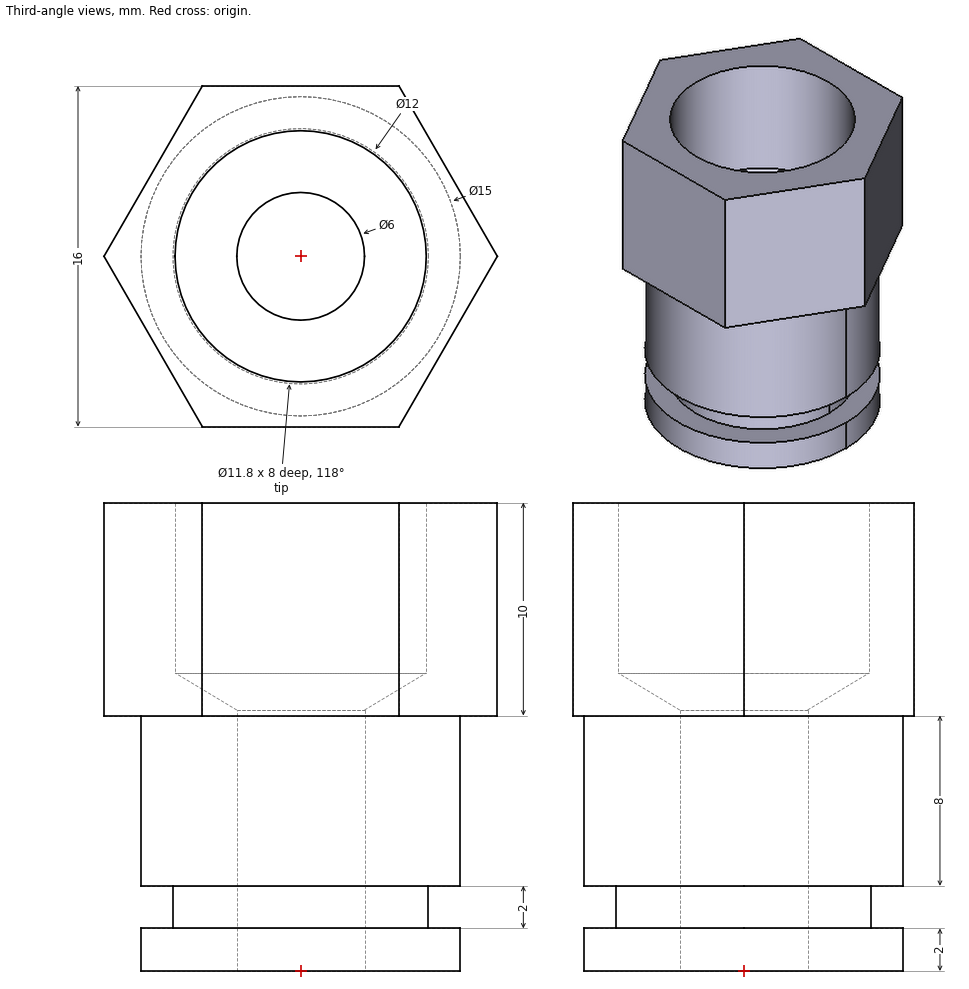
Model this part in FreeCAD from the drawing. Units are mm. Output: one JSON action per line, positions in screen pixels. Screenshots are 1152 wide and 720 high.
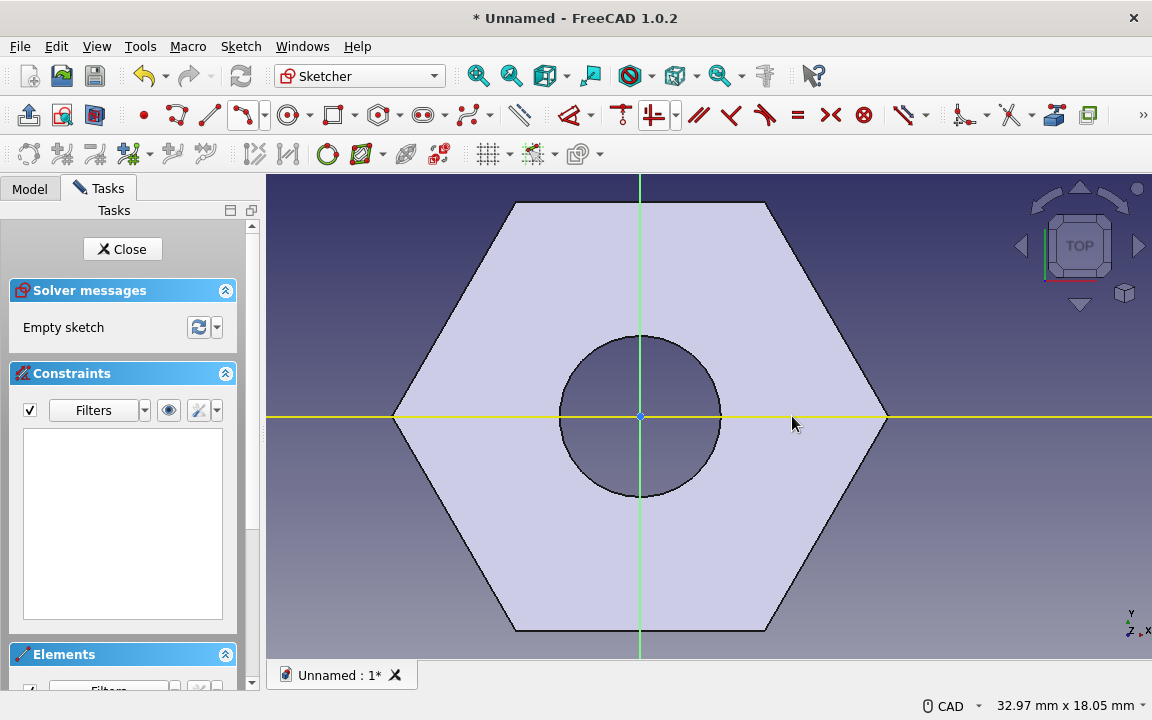
{"action": "left_click", "coordinate": [288, 116]}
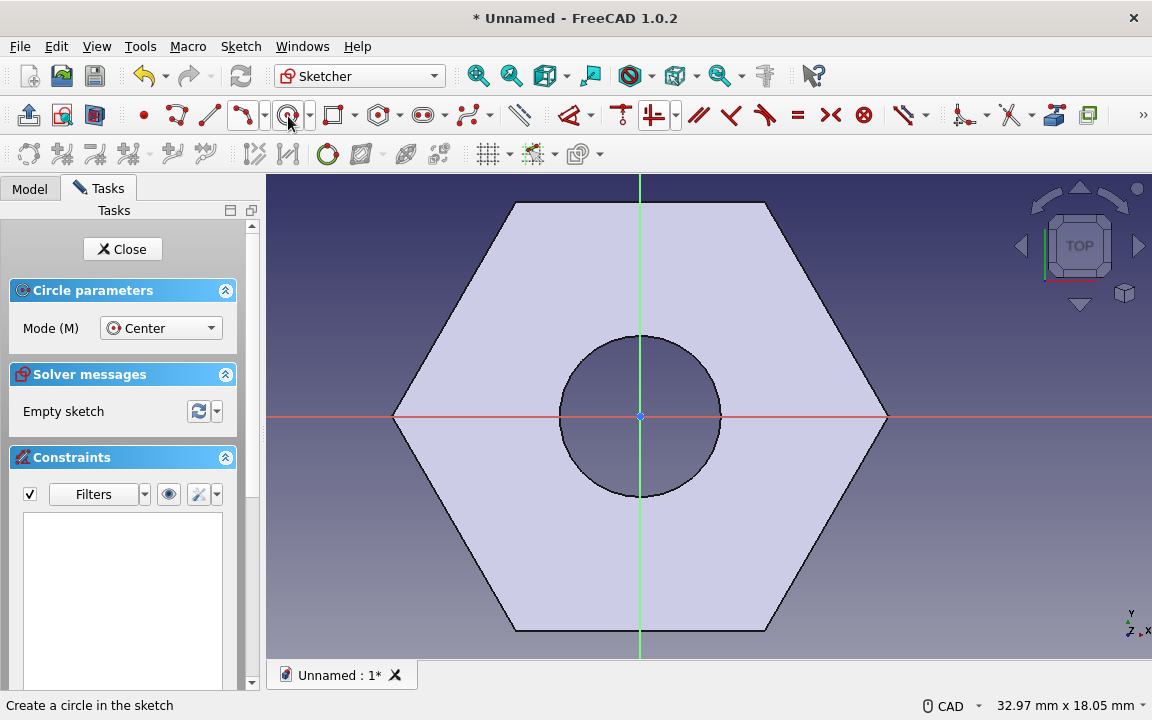
{"action": "left_click", "coordinate": [640, 416]}
{"action": "left_click", "coordinate": [752, 304]}
{"action": "key", "text": "Escape"}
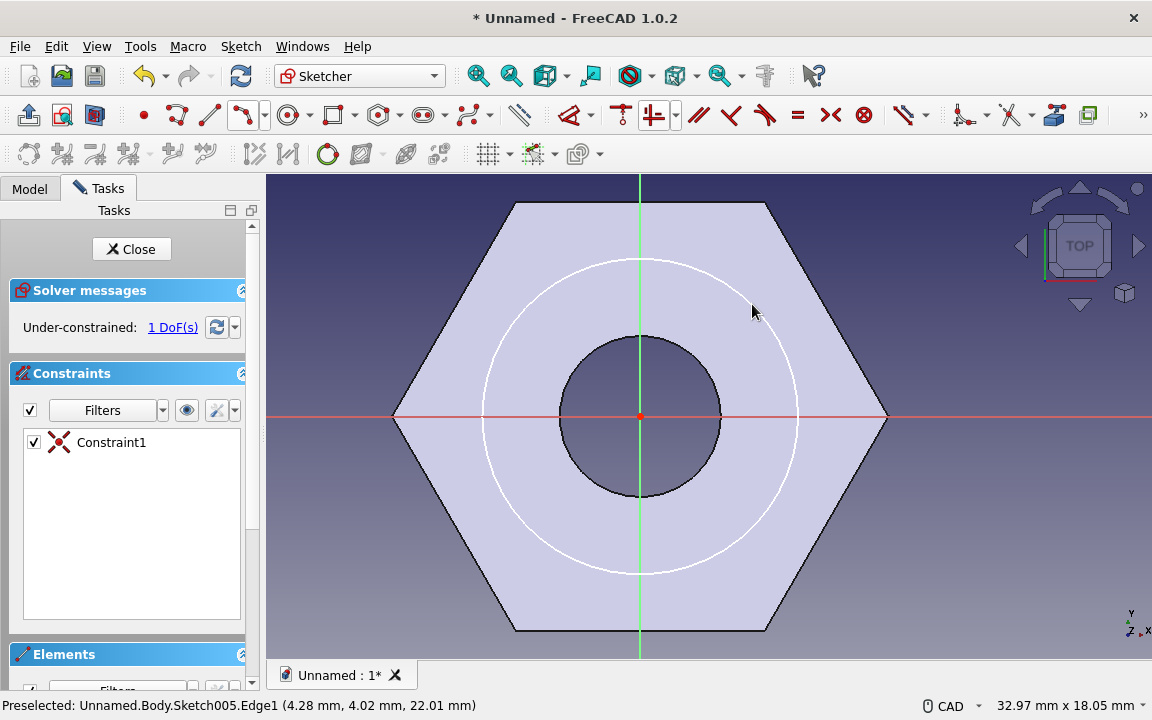
{"action": "key", "text": "d"}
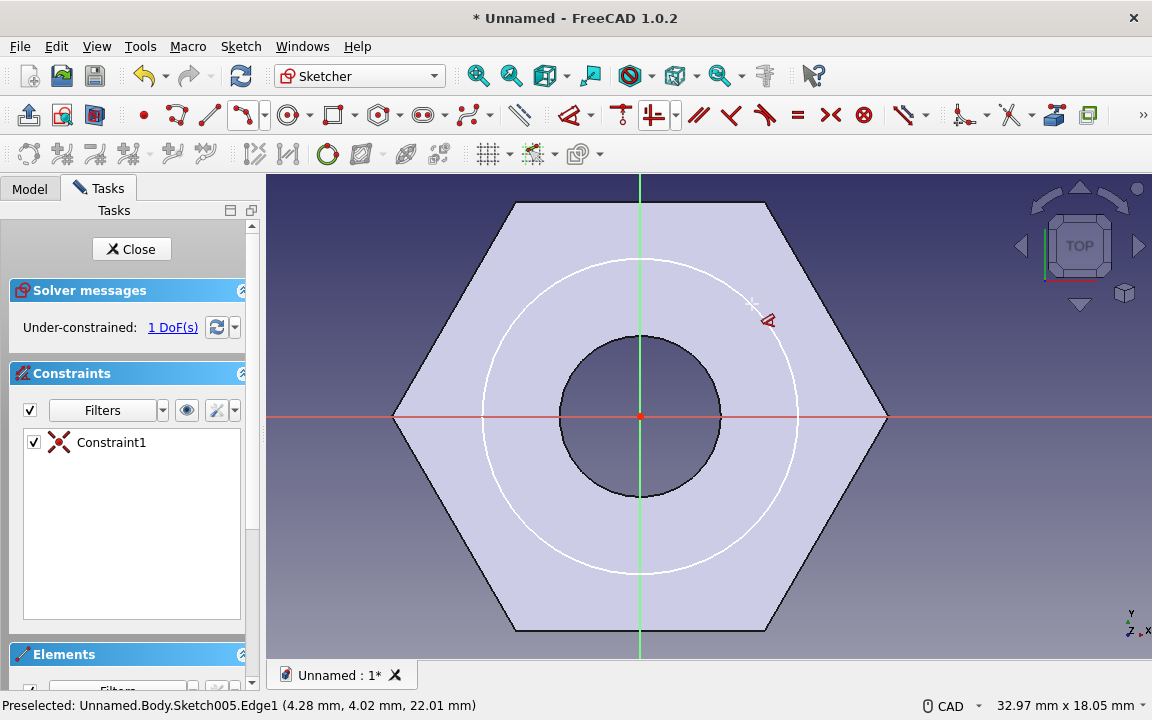
{"action": "left_click", "coordinate": [752, 305]}
{"action": "left_click", "coordinate": [775, 282]}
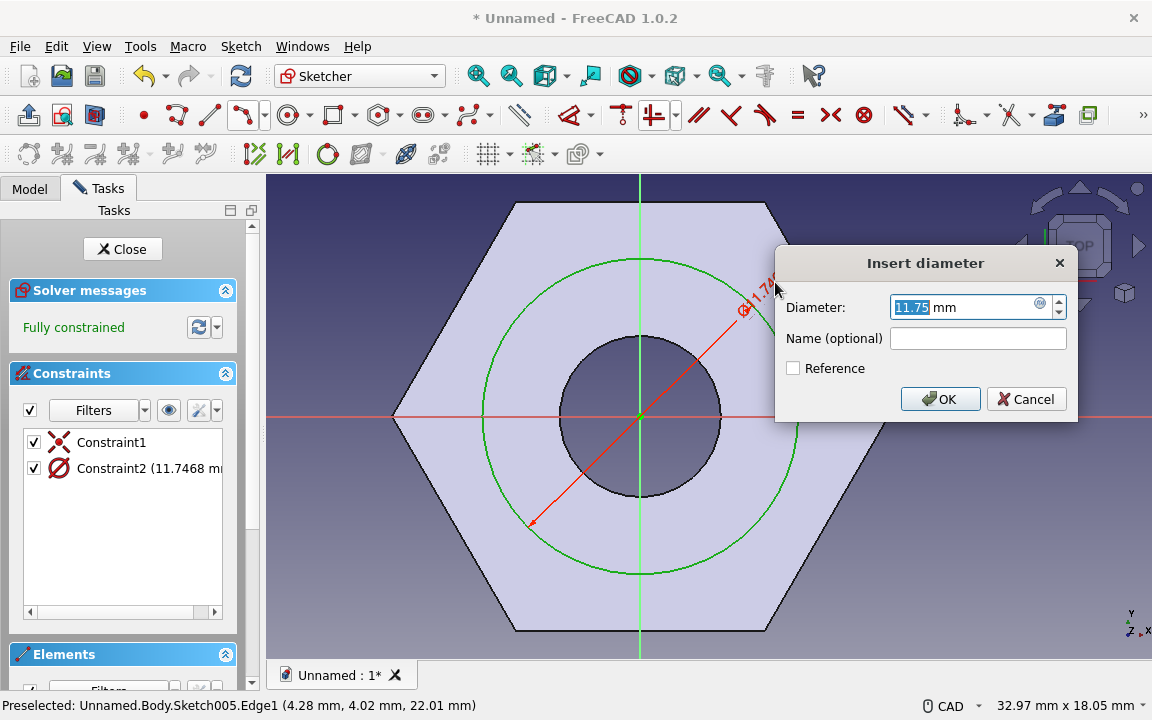
{"action": "type", "text": "11.8"}
{"action": "key", "text": "Return"}
{"action": "key", "text": "Escape"}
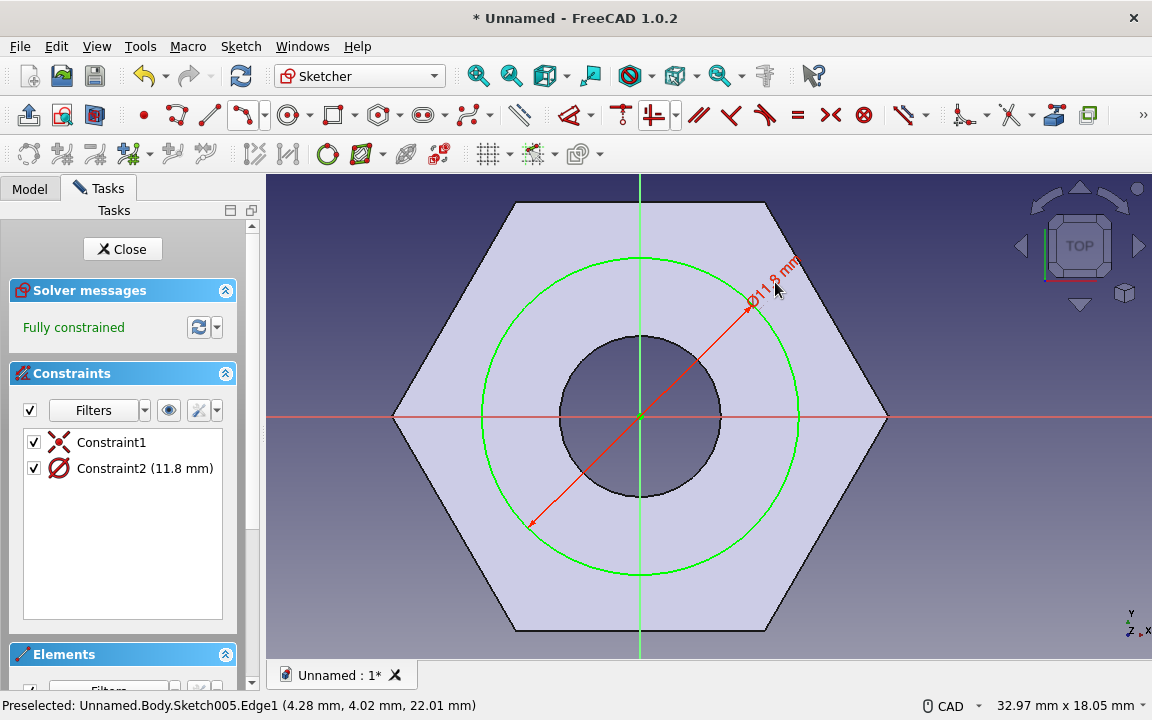
{"action": "left_click", "coordinate": [123, 249]}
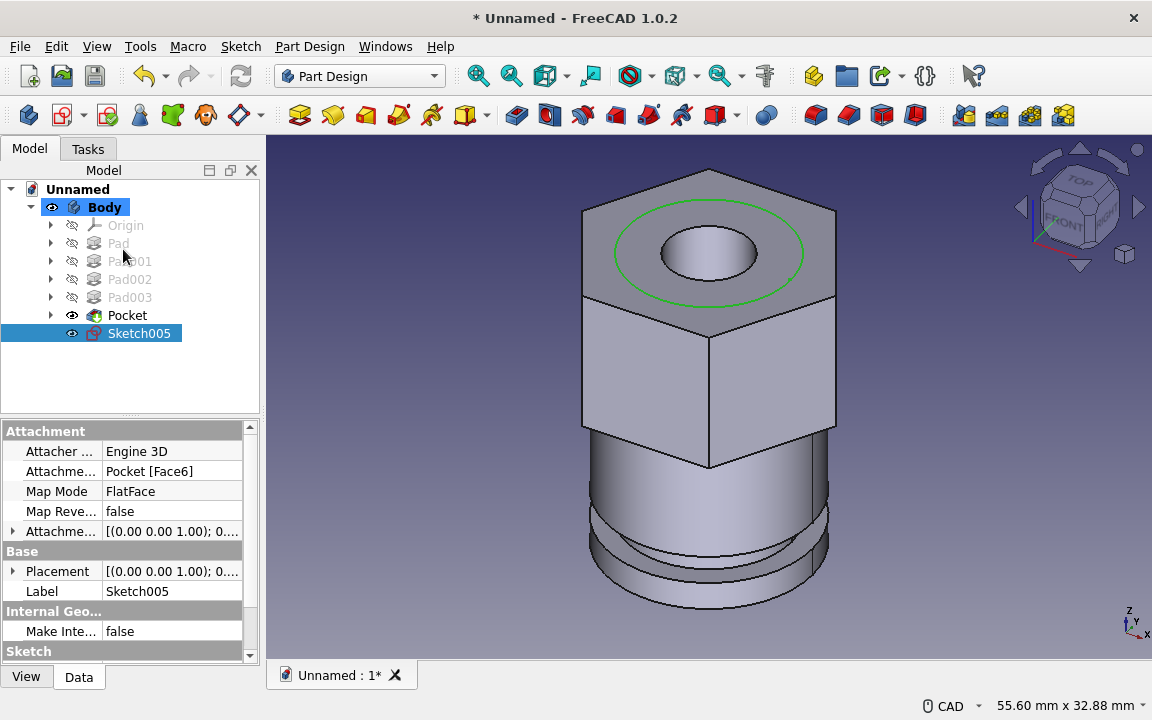
{"action": "left_click", "coordinate": [550, 116]}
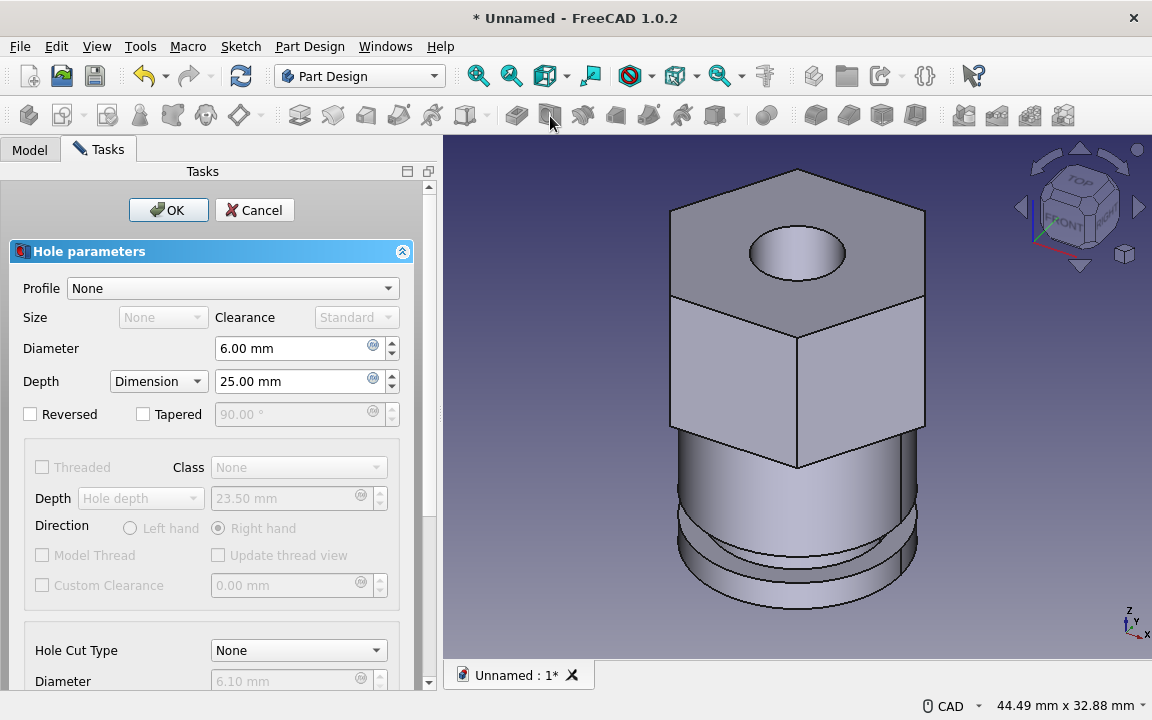
{"action": "triple_click", "coordinate": [300, 348]}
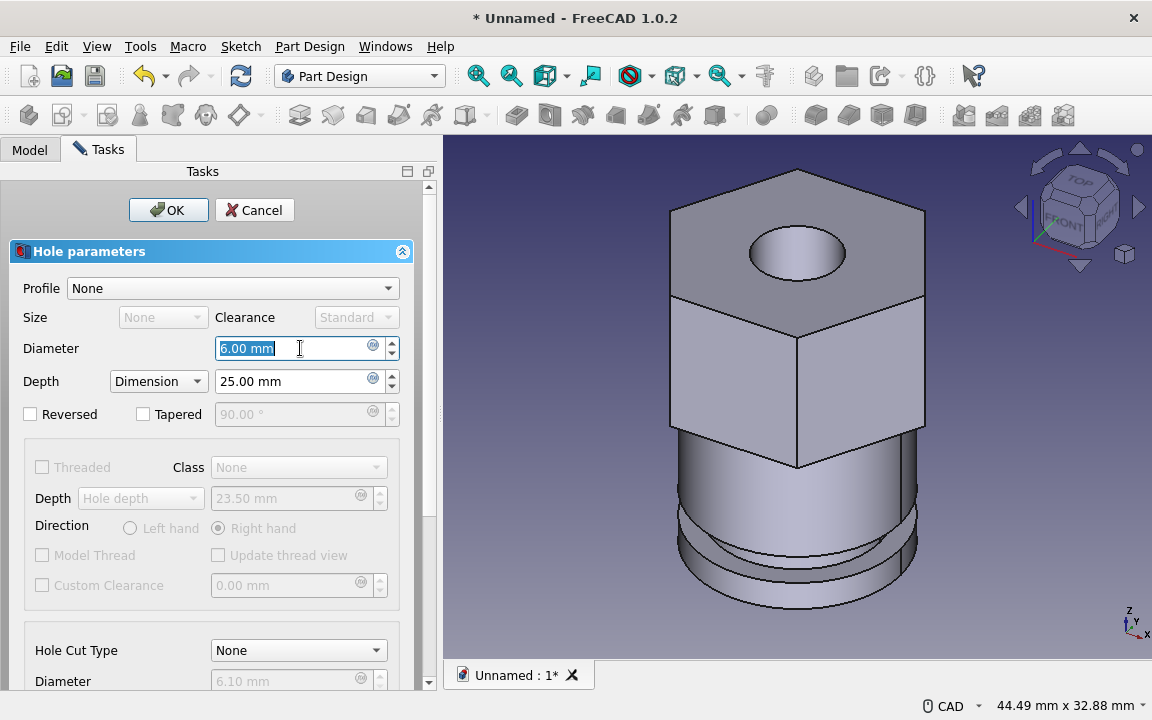
{"action": "type", "text": "11.8"}
{"action": "key", "text": "Tab"}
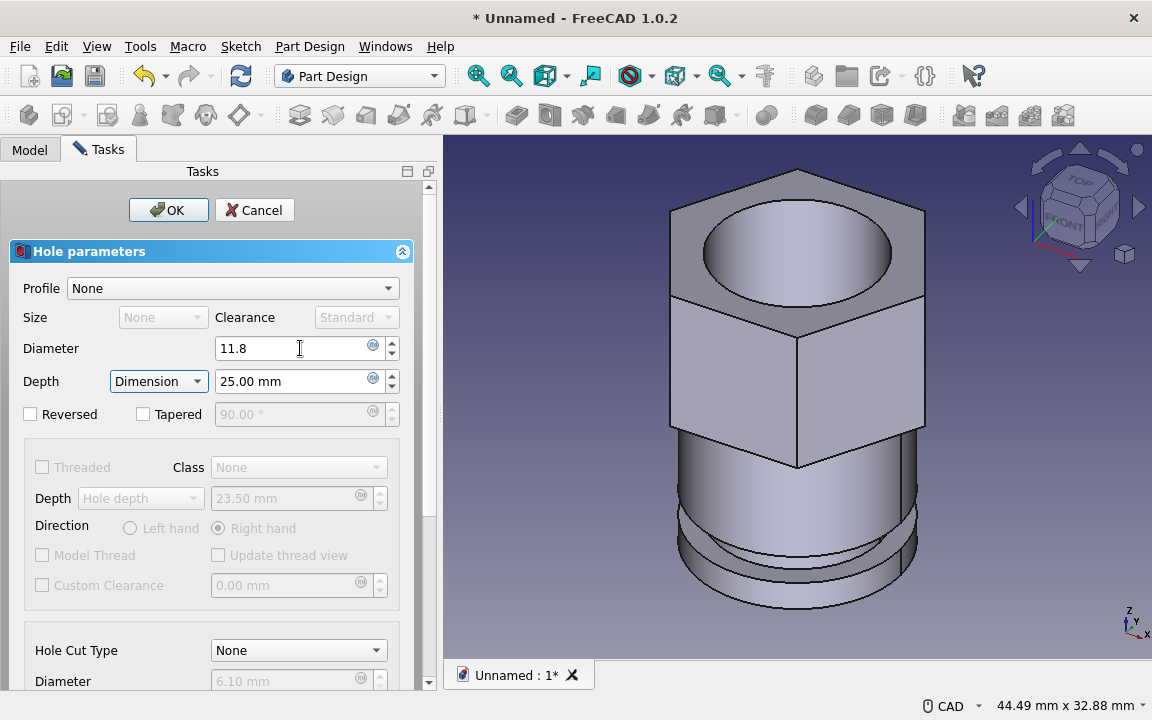
{"action": "triple_click", "coordinate": [300, 382]}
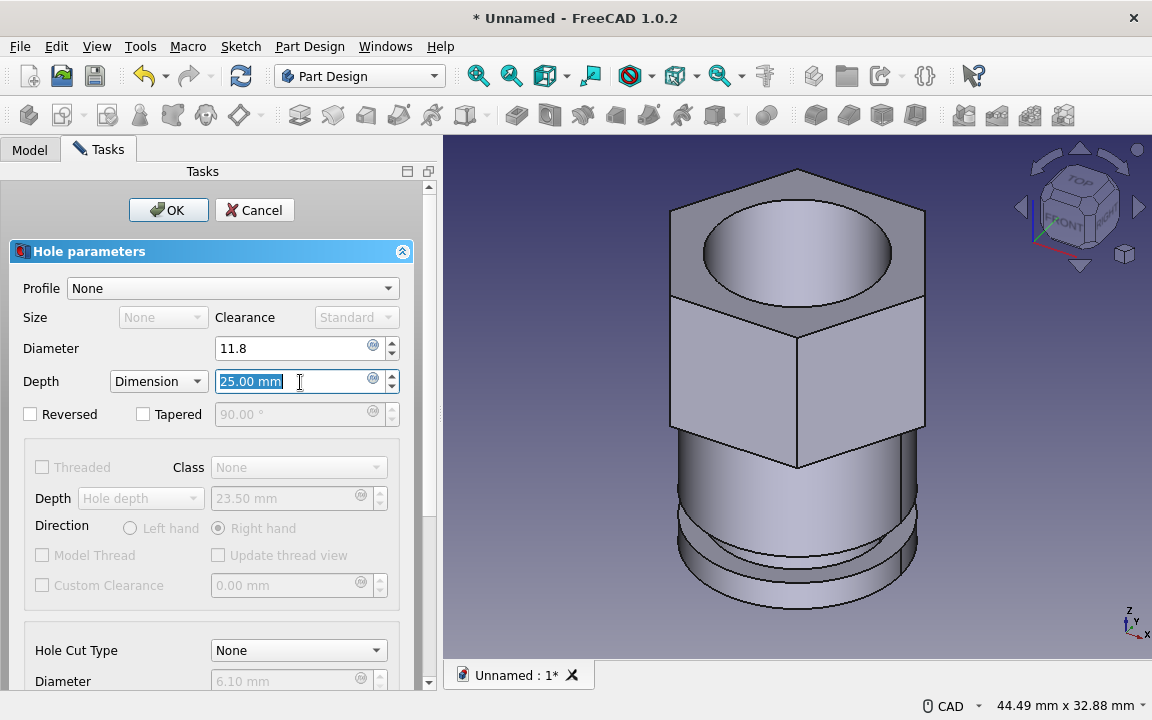
{"action": "type", "text": "8"}
{"action": "key", "text": "Tab"}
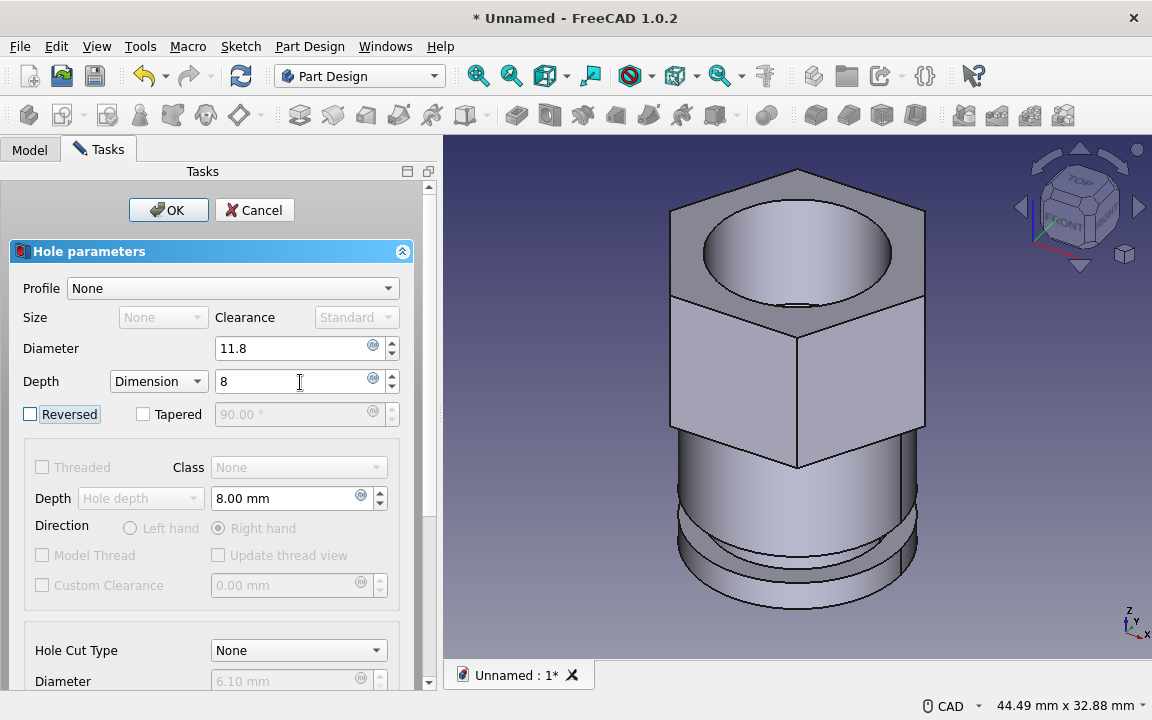
{"action": "left_click", "coordinate": [169, 210]}